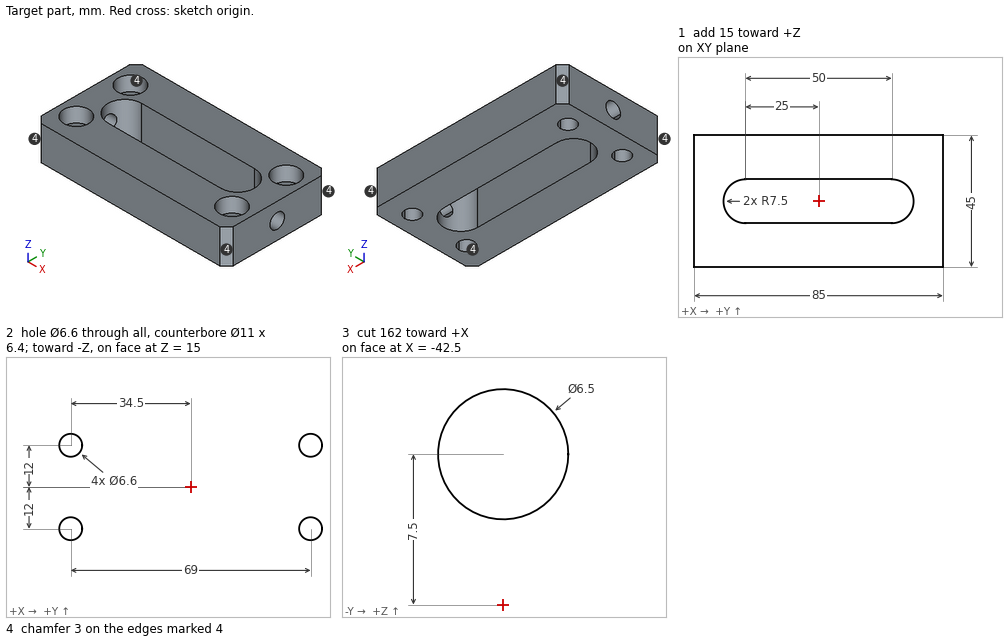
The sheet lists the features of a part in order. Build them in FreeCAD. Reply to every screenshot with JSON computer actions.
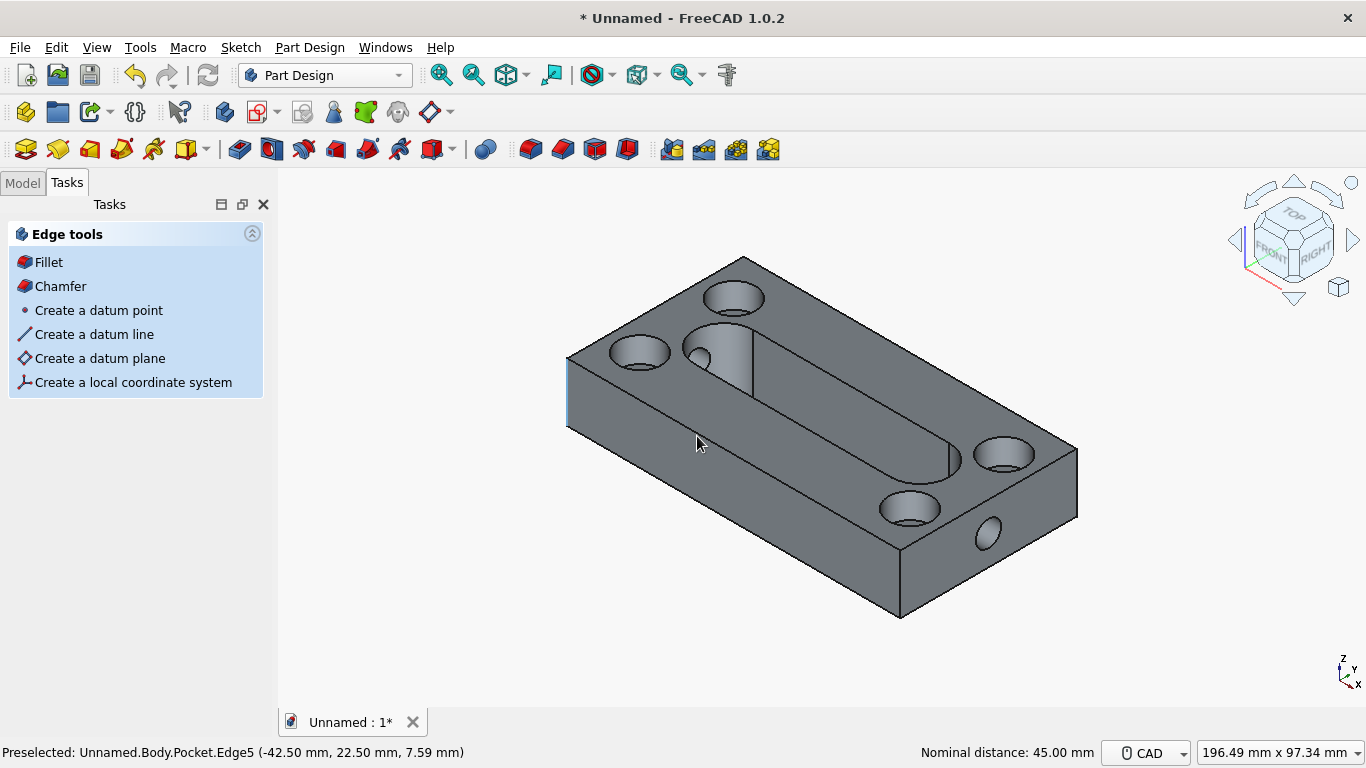
{"action": "left_click", "coordinate": [900, 583], "text": "ctrl"}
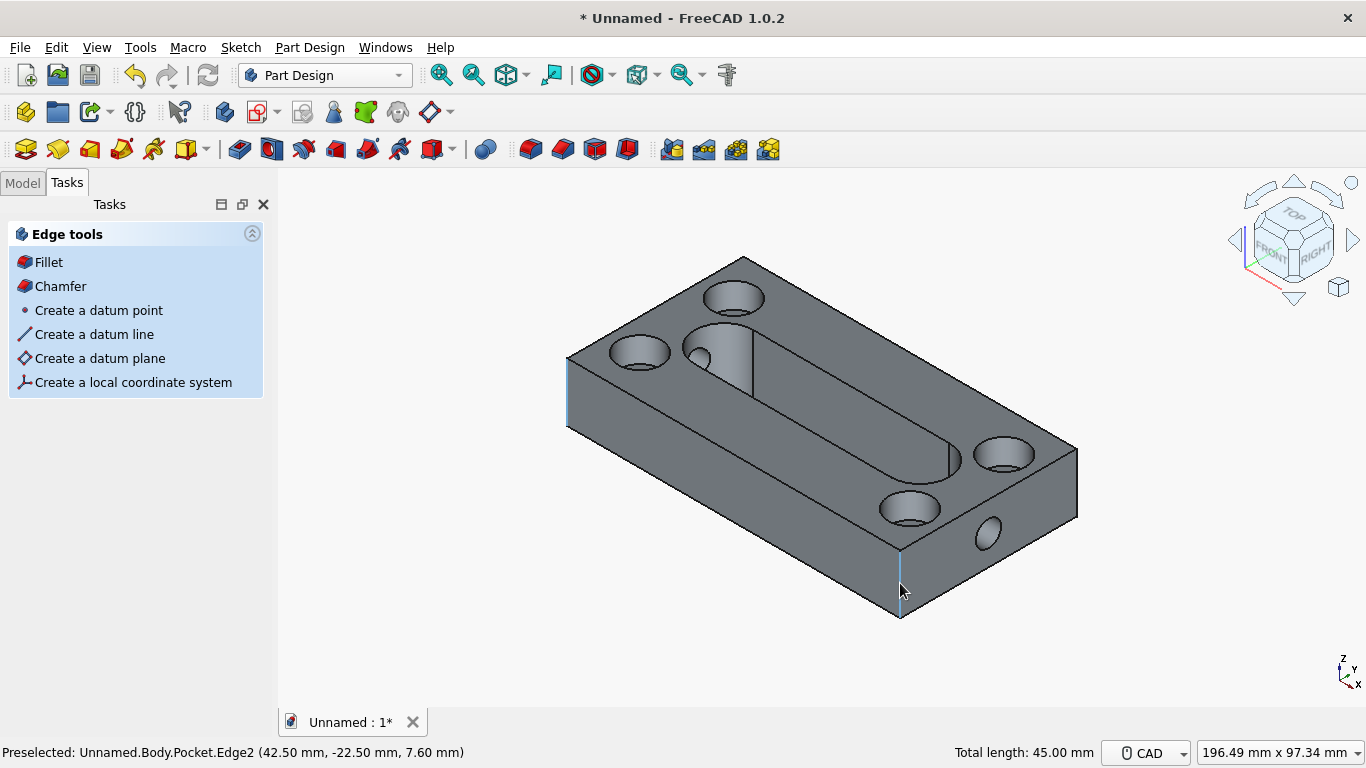
{"action": "key", "text": "2"}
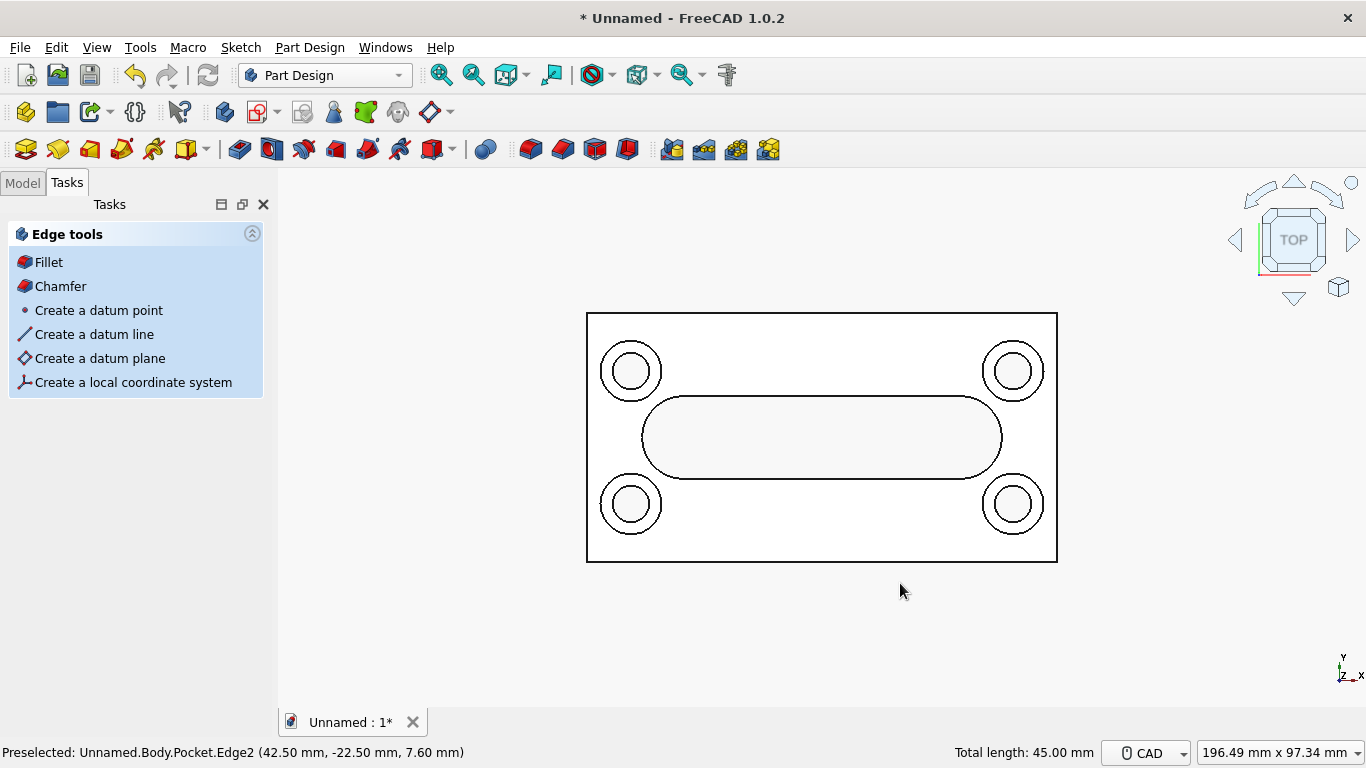
{"action": "key", "text": "1"}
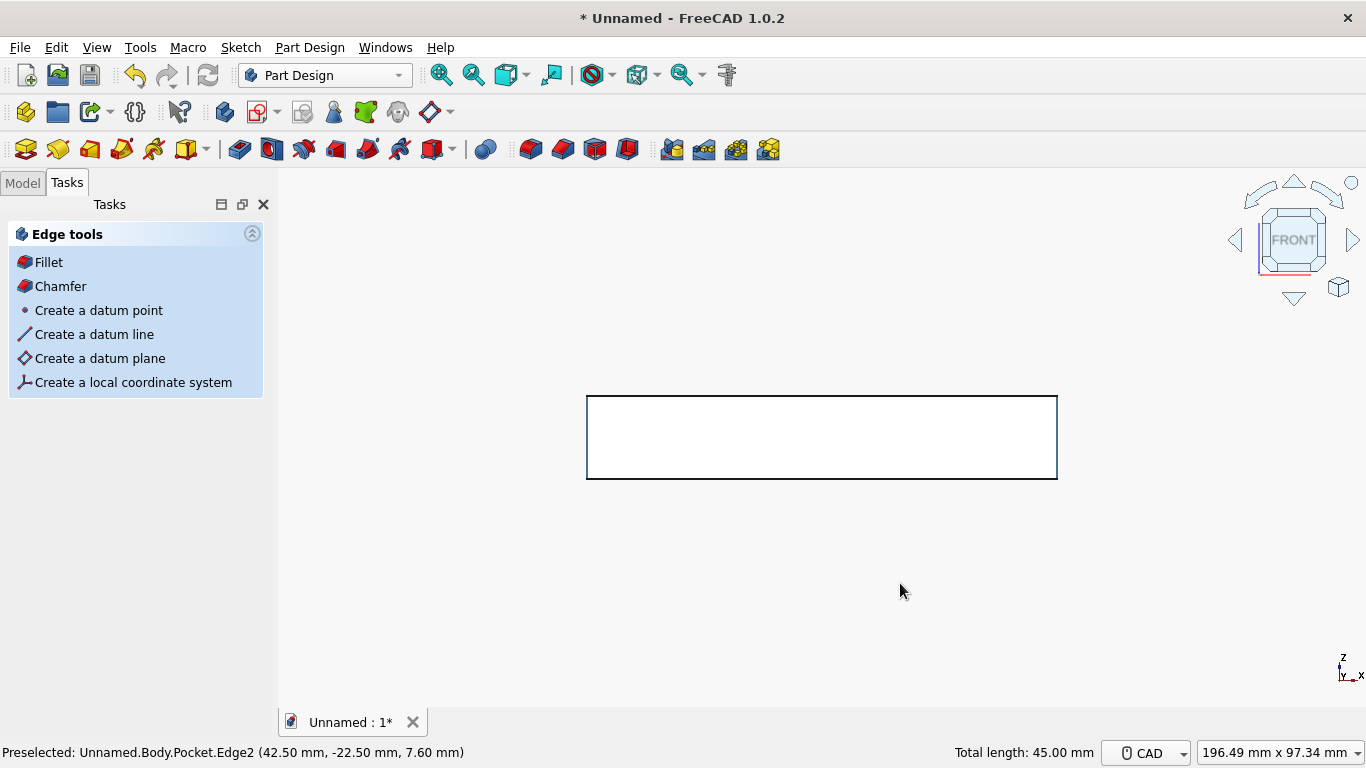
{"action": "left_click", "coordinate": [442, 76]}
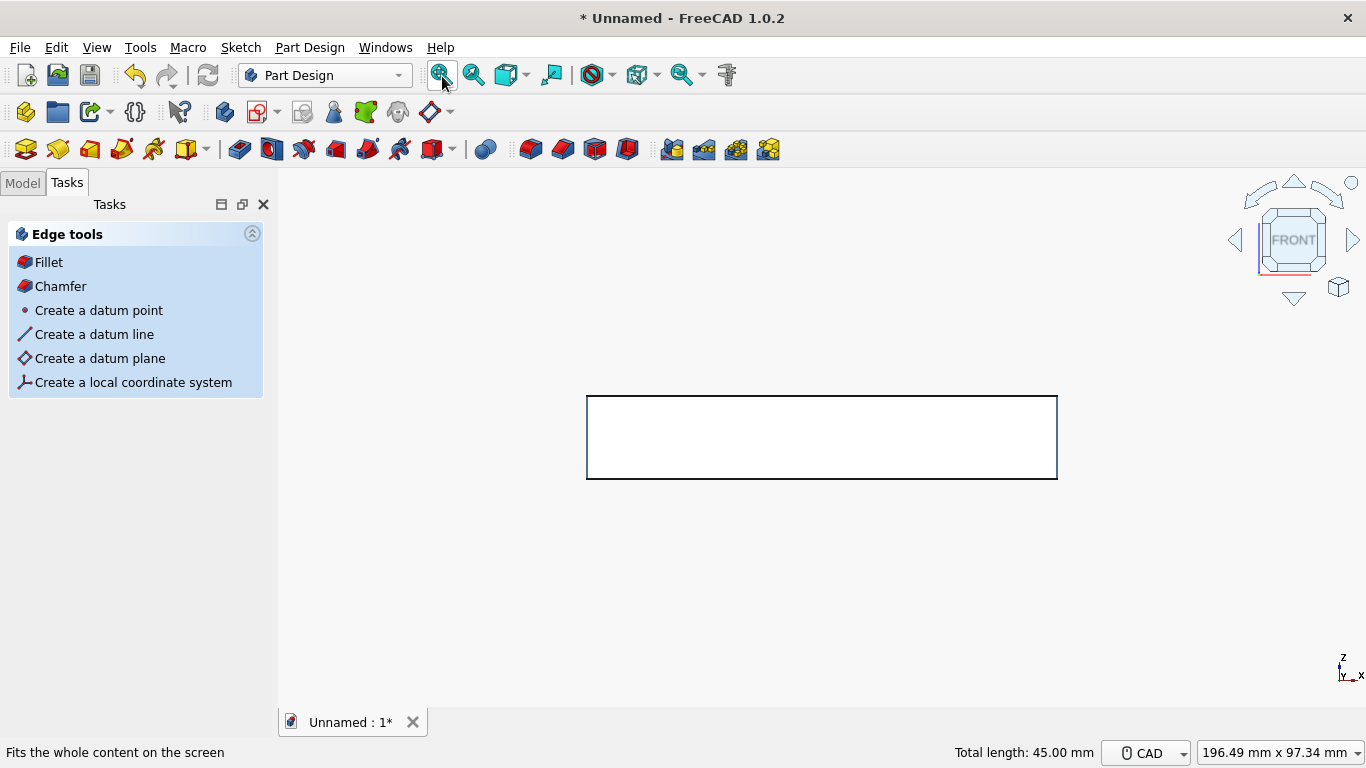
{"action": "key", "text": "3"}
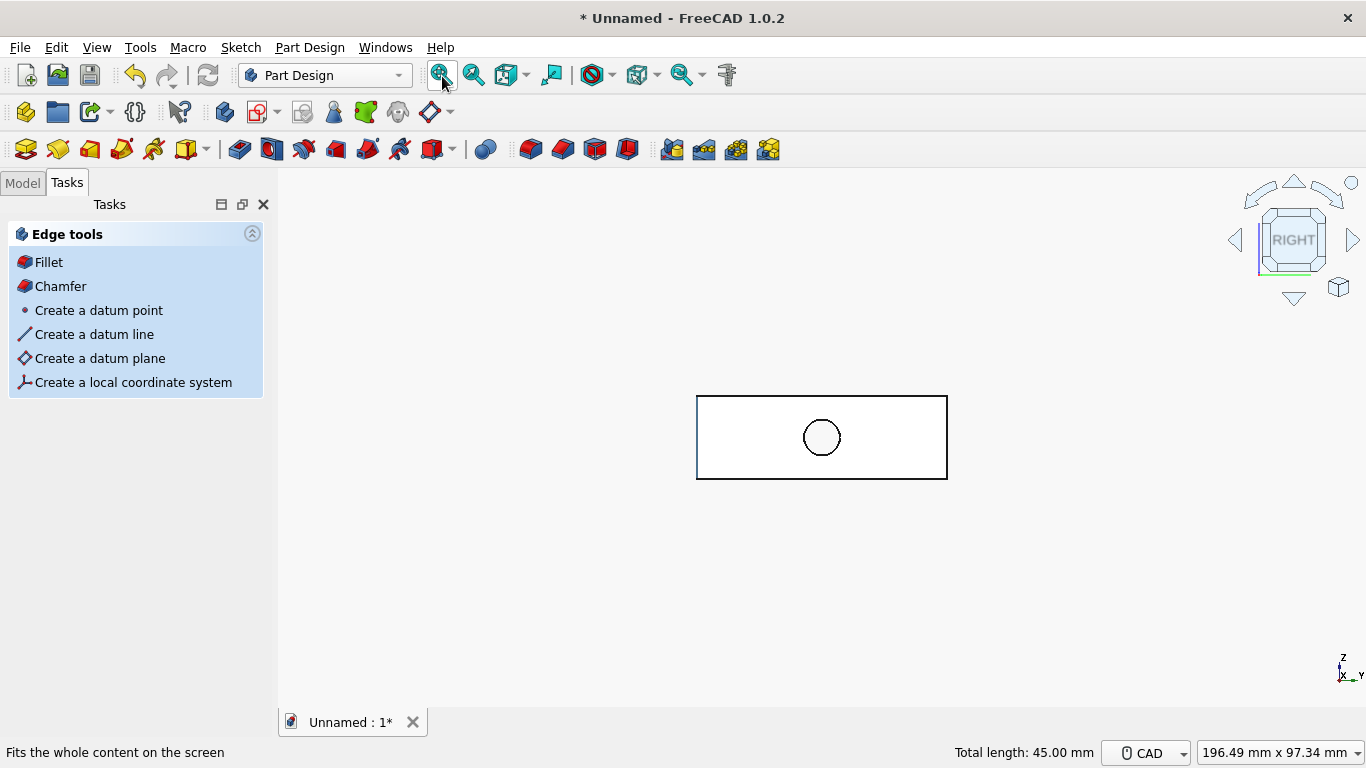
{"action": "left_click", "coordinate": [442, 76]}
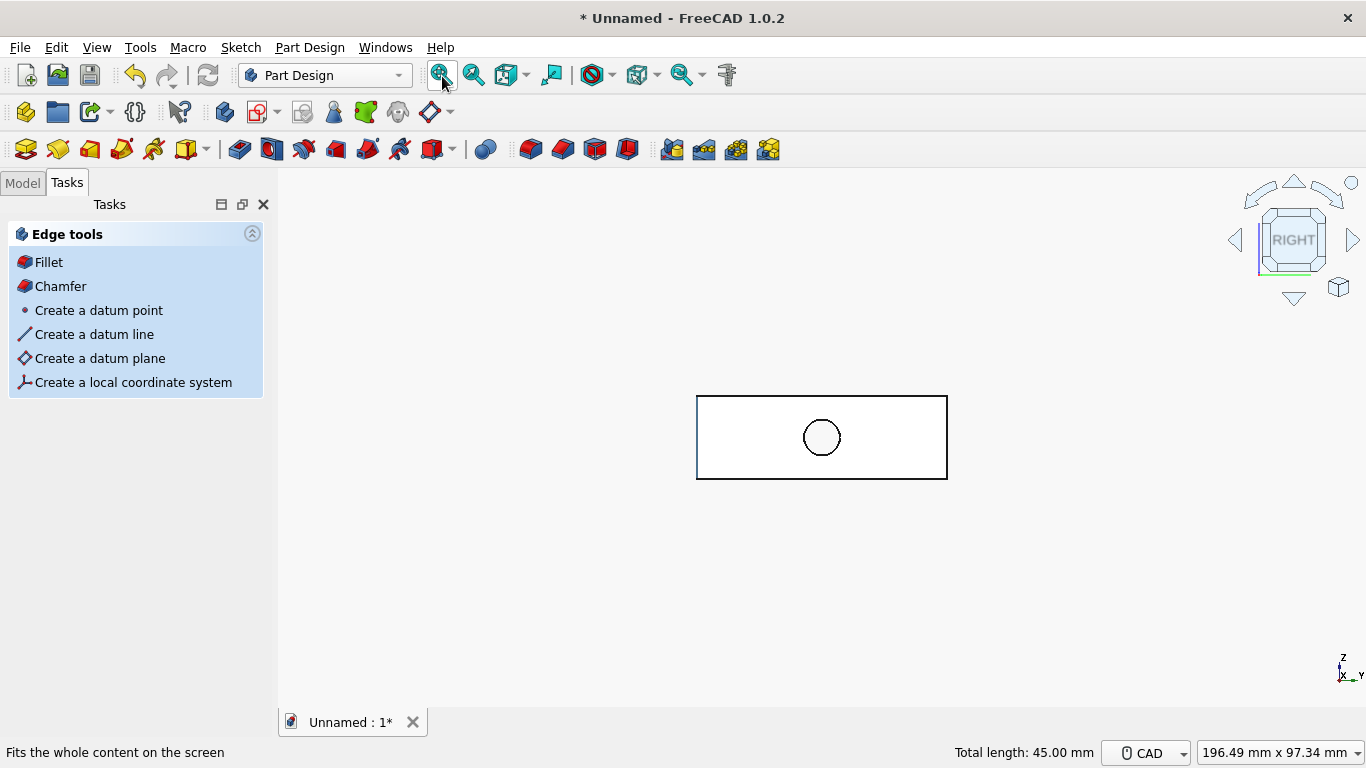
{"action": "left_click", "coordinate": [947, 436], "text": "ctrl"}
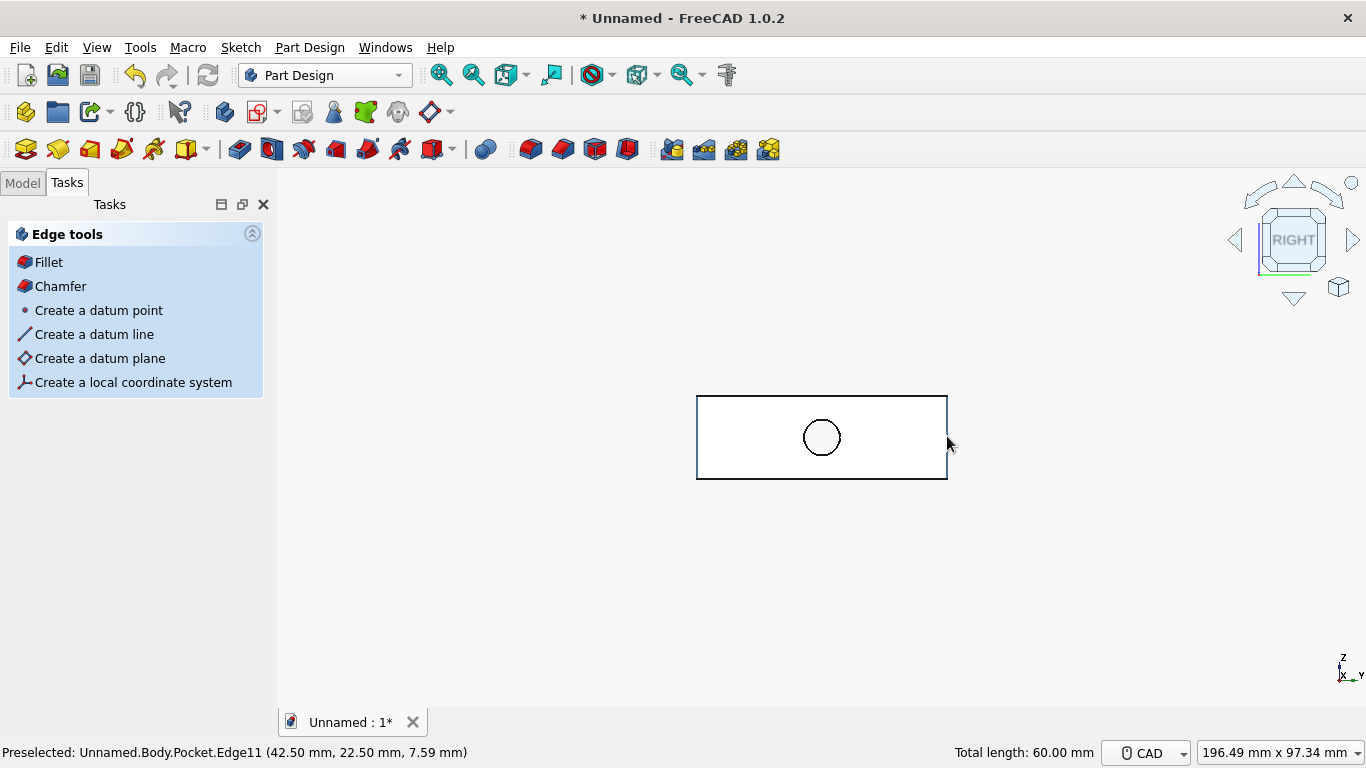
{"action": "left_click", "coordinate": [564, 150]}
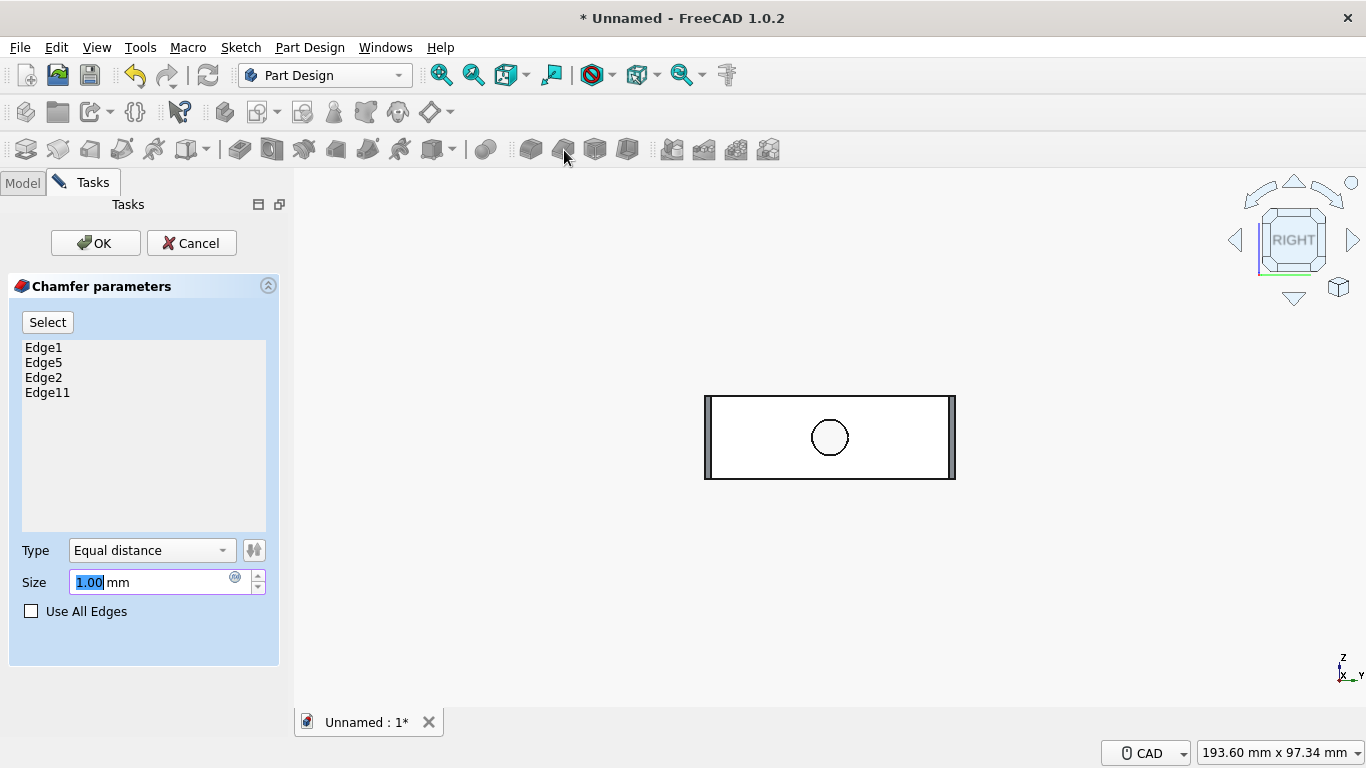
{"action": "type", "text": "3"}
{"action": "key", "text": "Tab"}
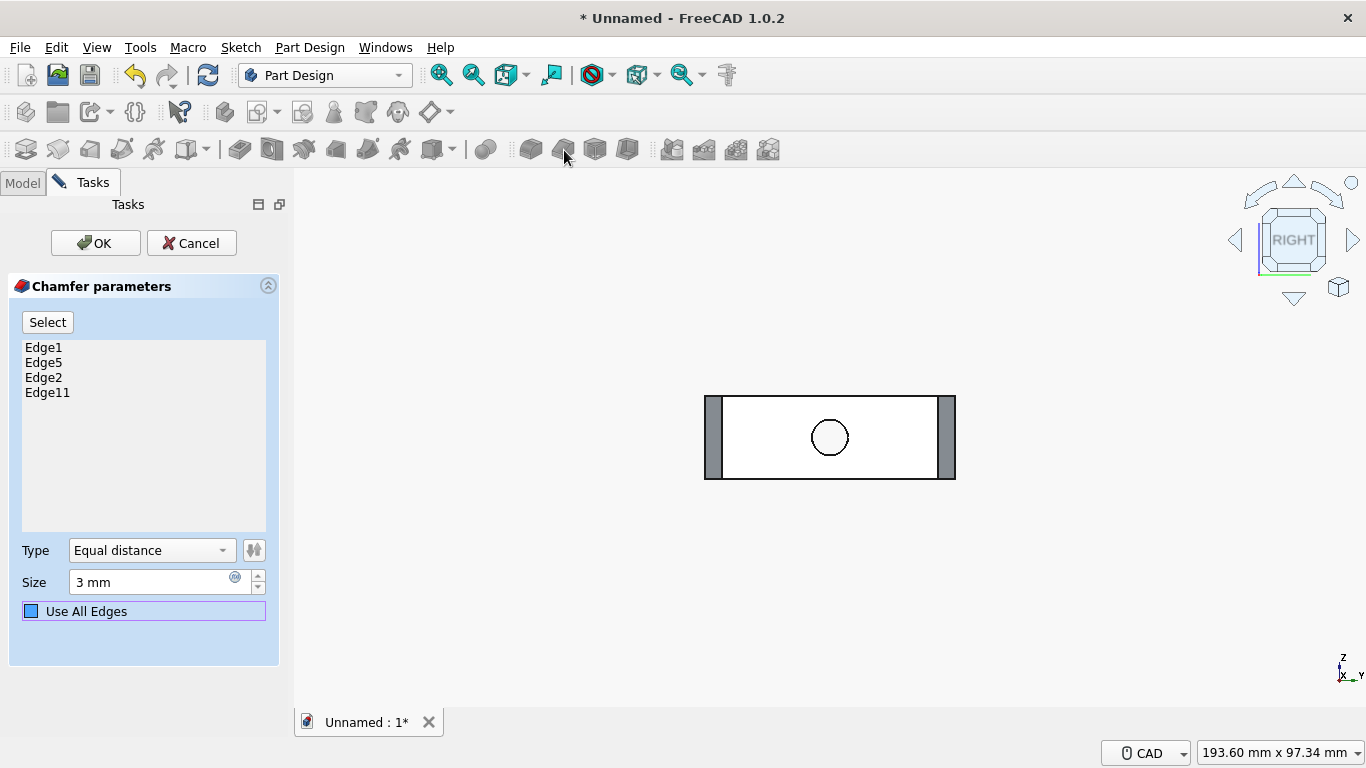
{"action": "left_click", "coordinate": [96, 243]}